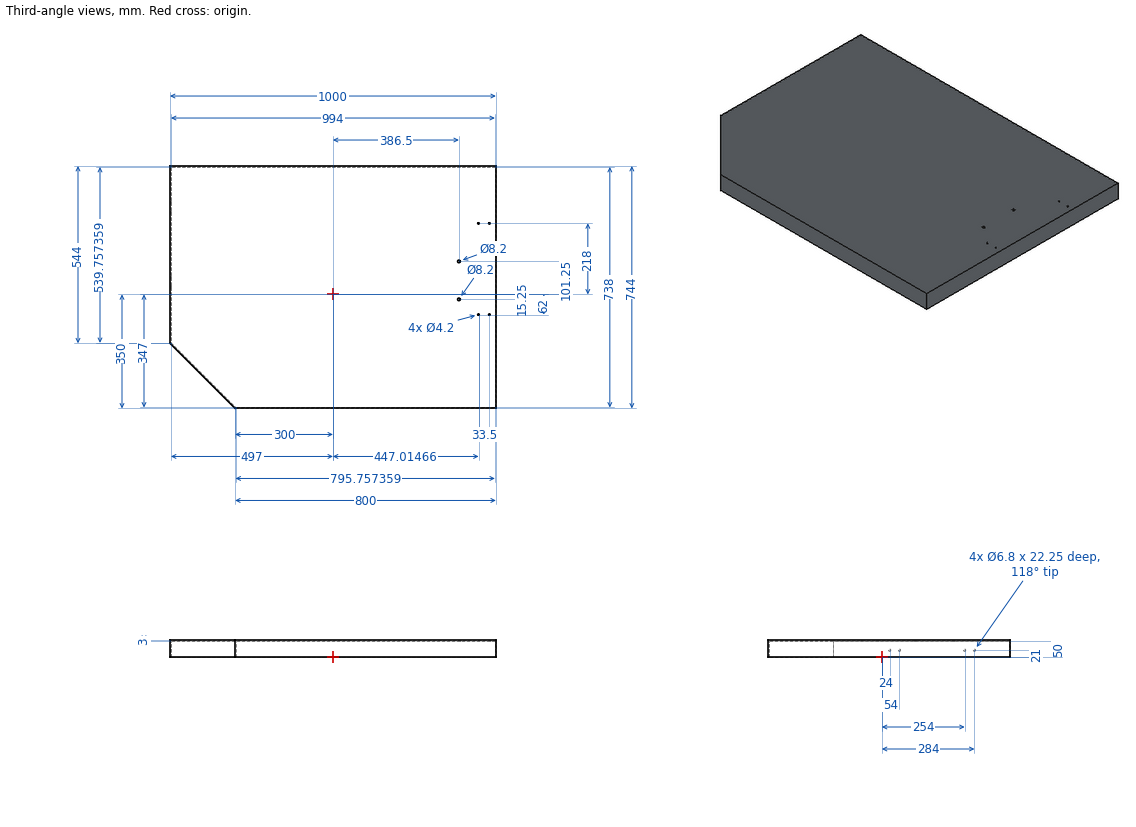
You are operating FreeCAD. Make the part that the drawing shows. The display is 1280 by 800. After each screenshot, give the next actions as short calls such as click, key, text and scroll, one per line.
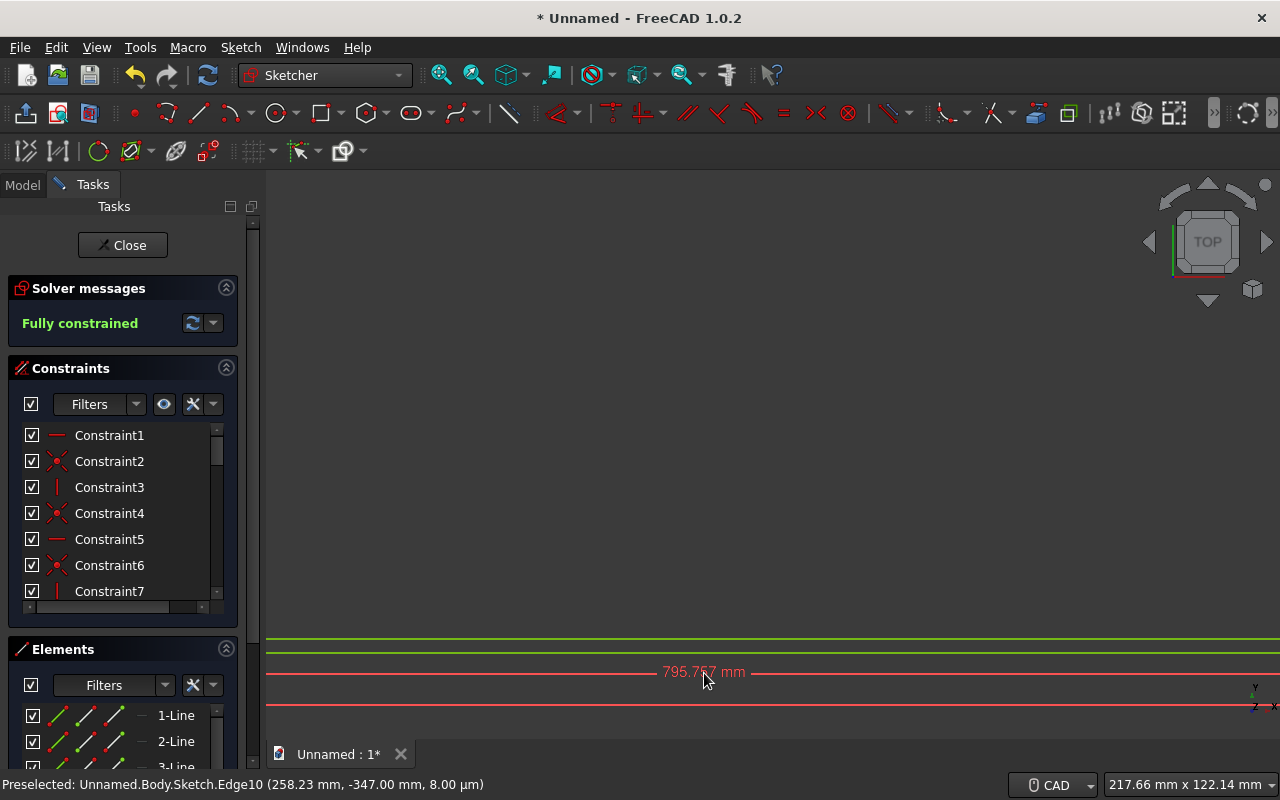
click(123, 245)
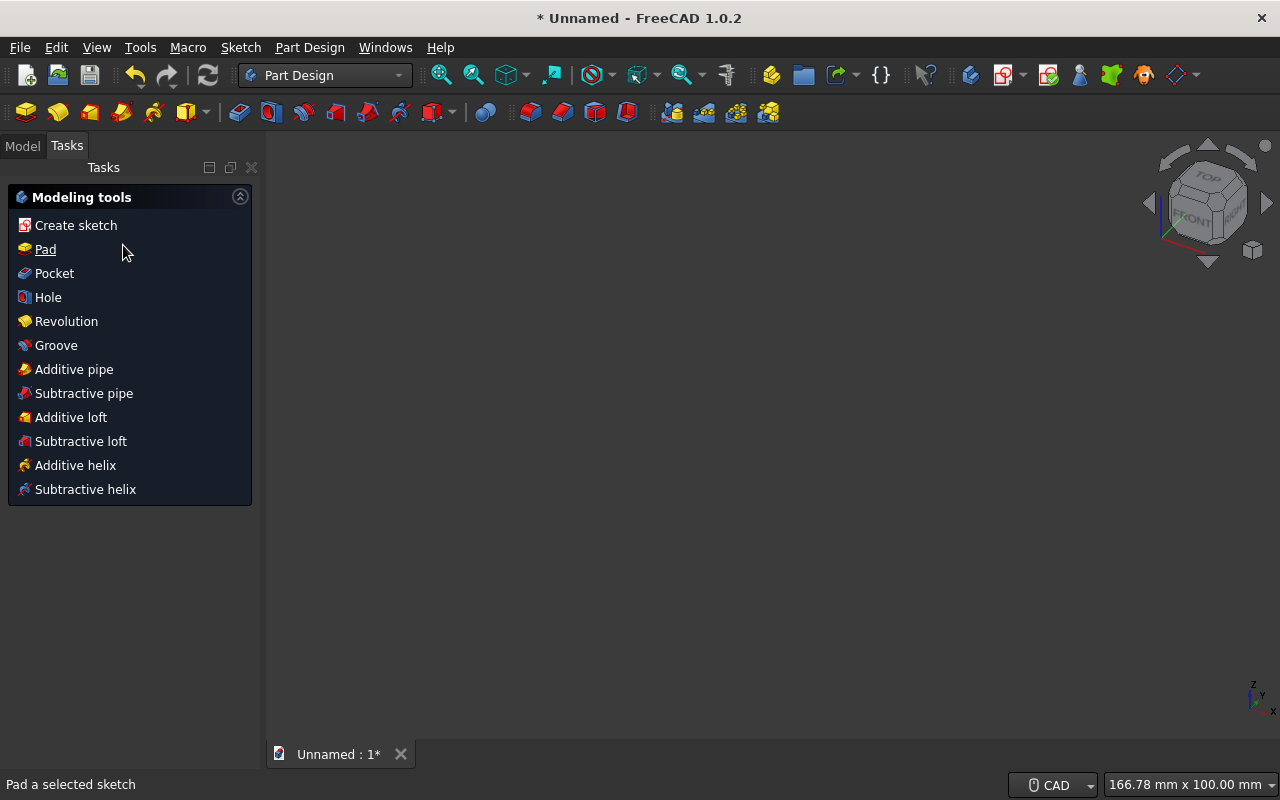
click(26, 112)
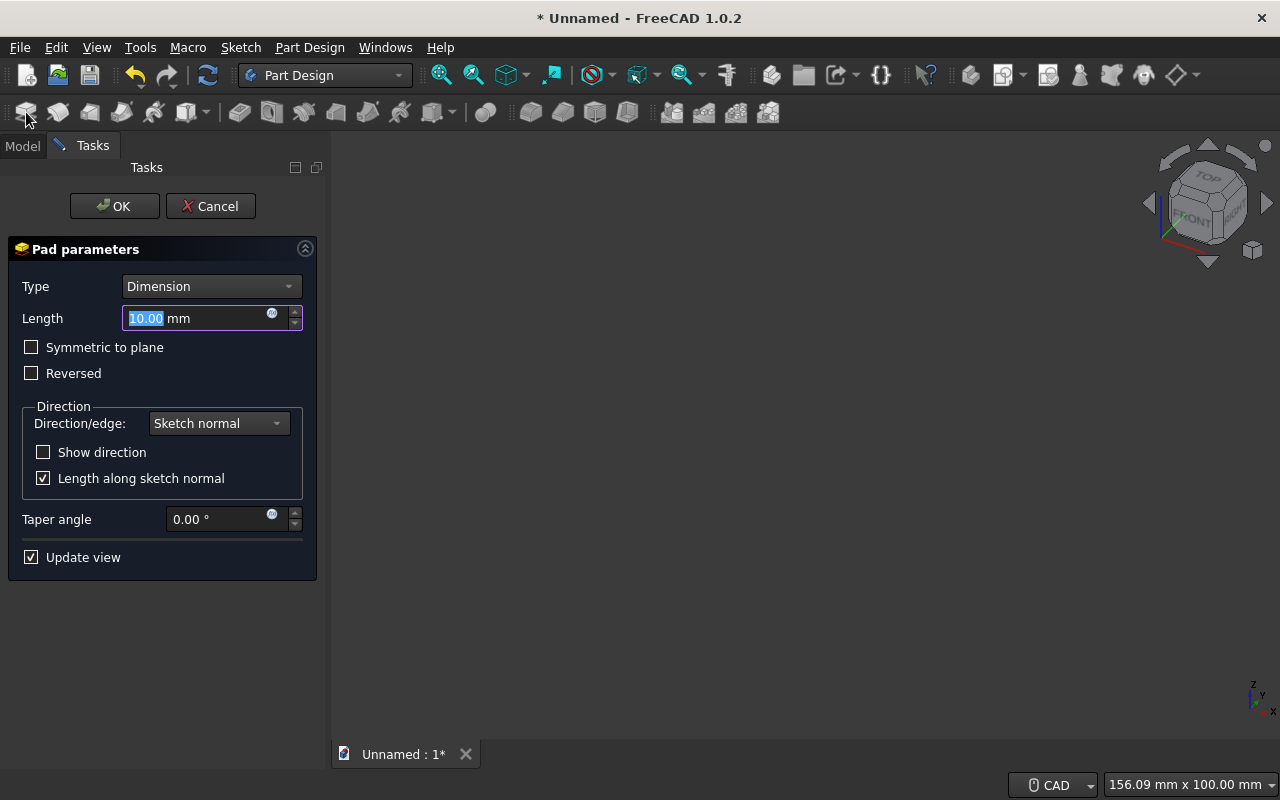
text(50)
key(Tab)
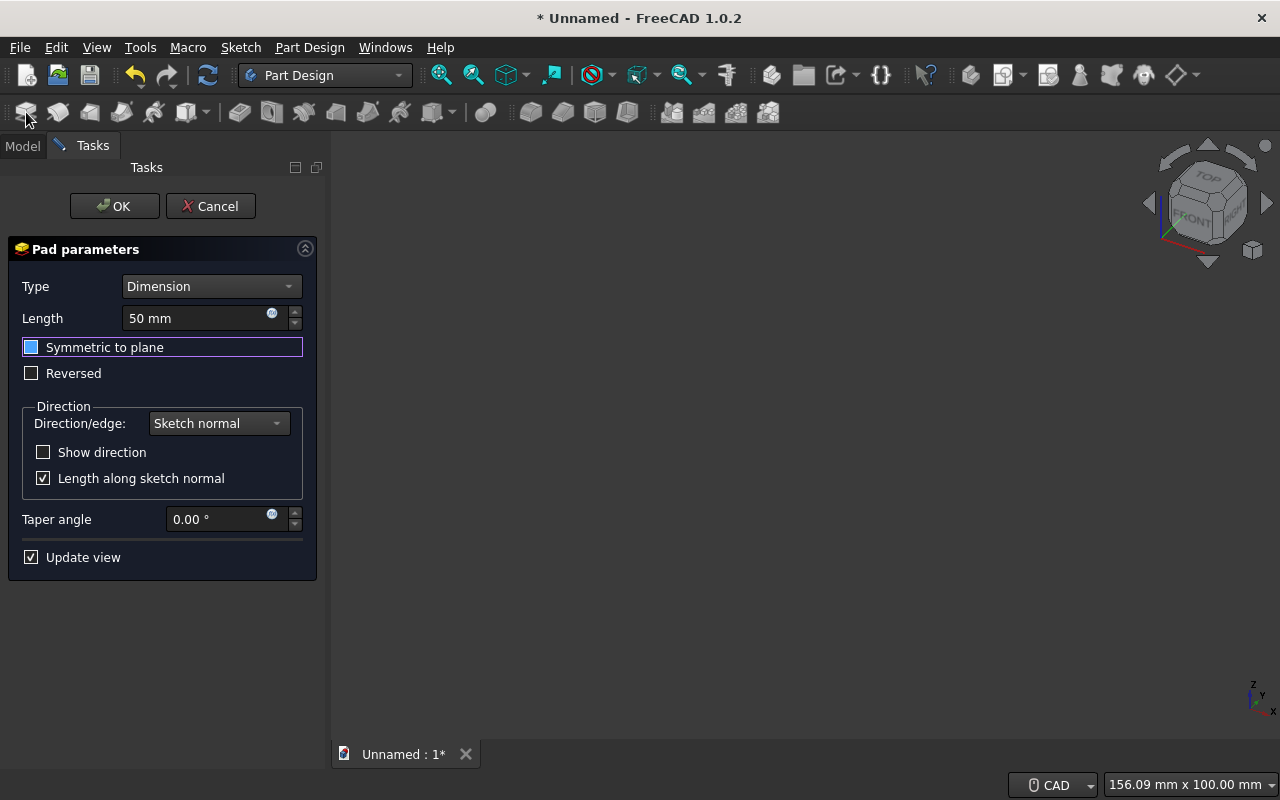
click(115, 206)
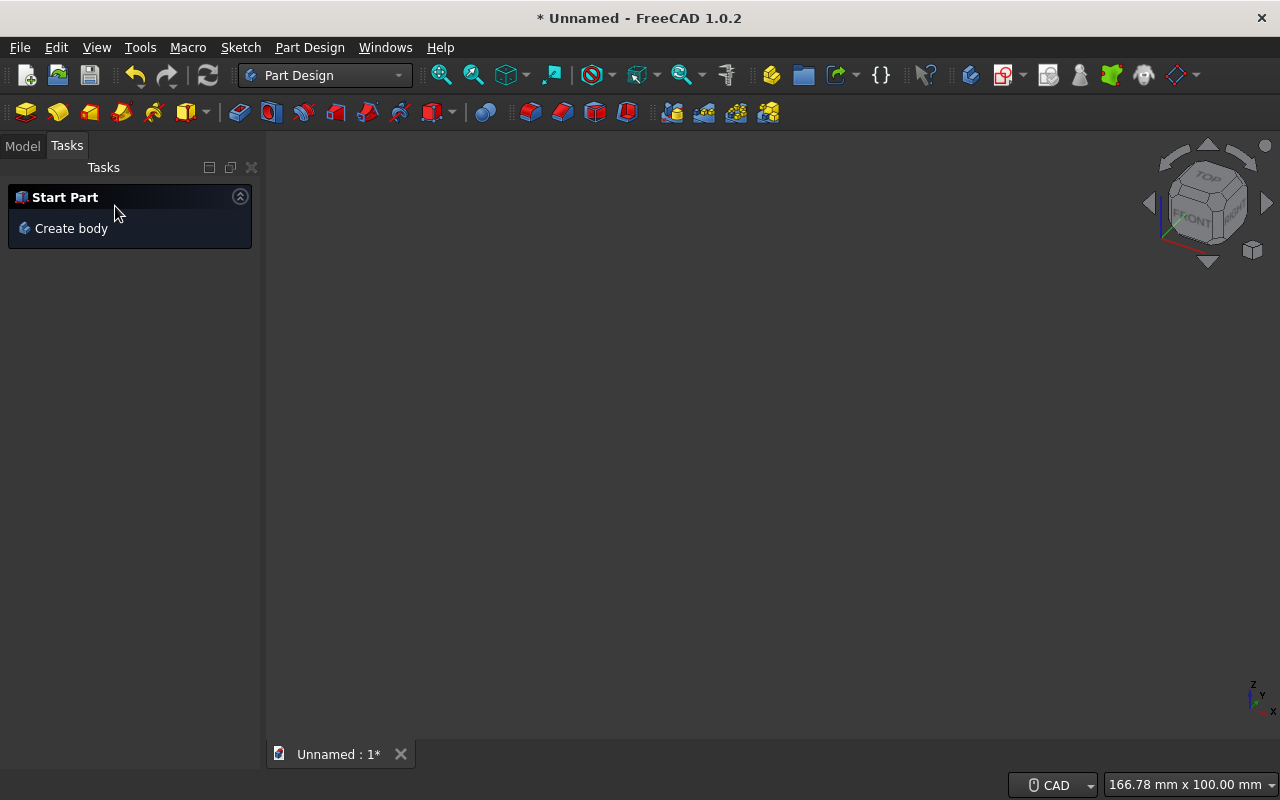
click(442, 76)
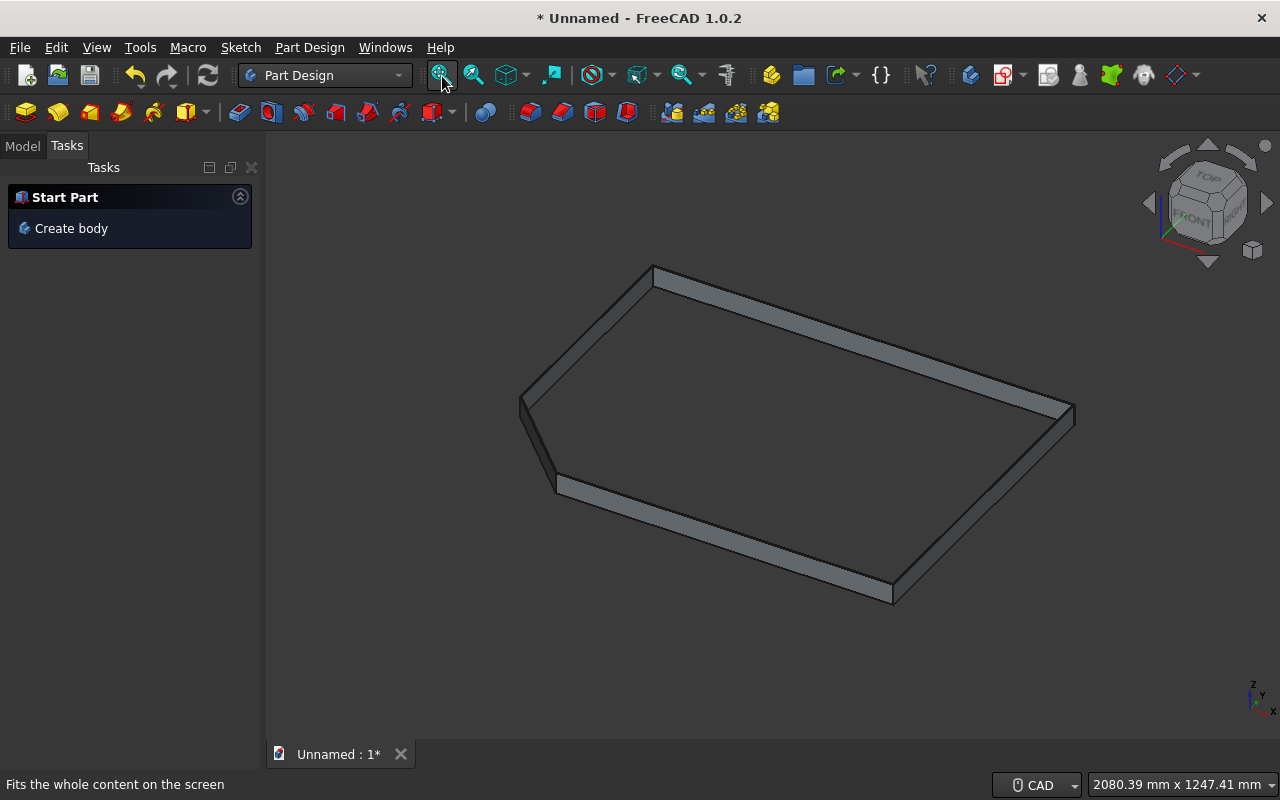
scroll(544, 447, up, 15)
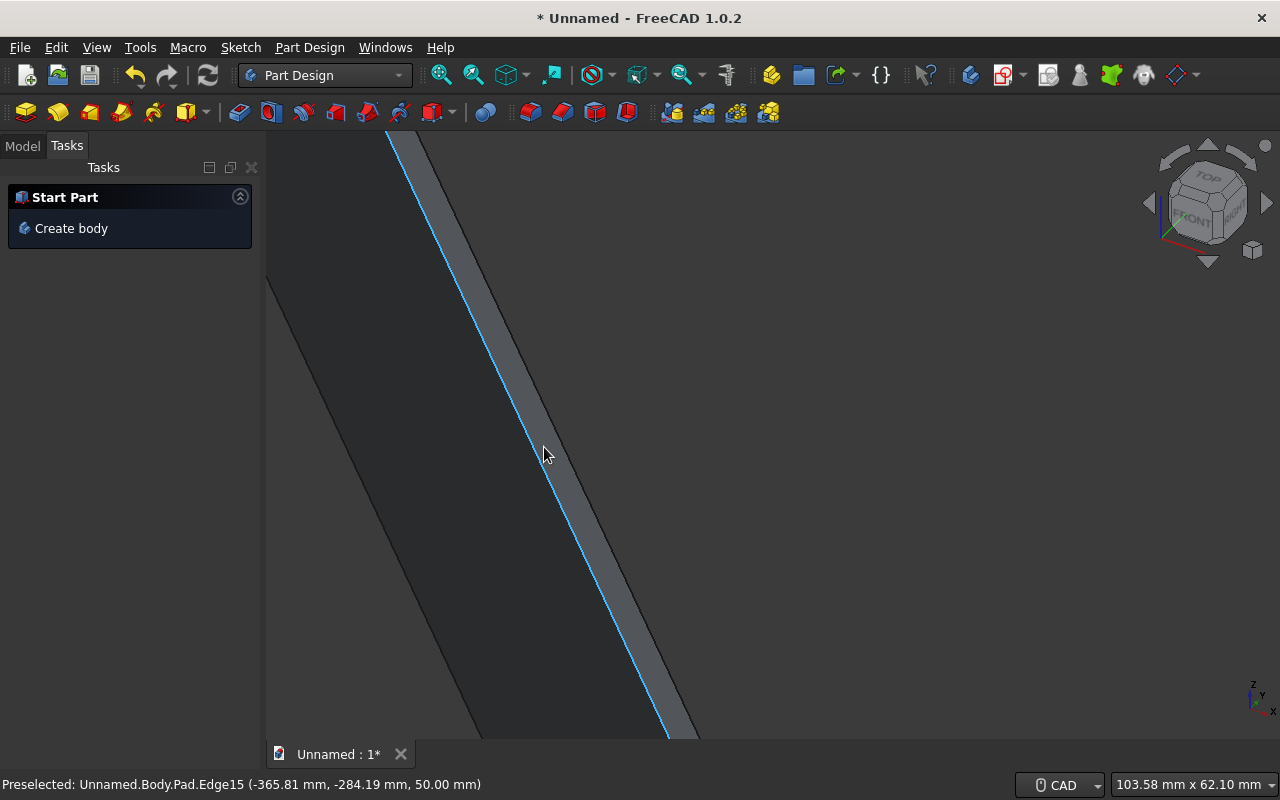
click(442, 76)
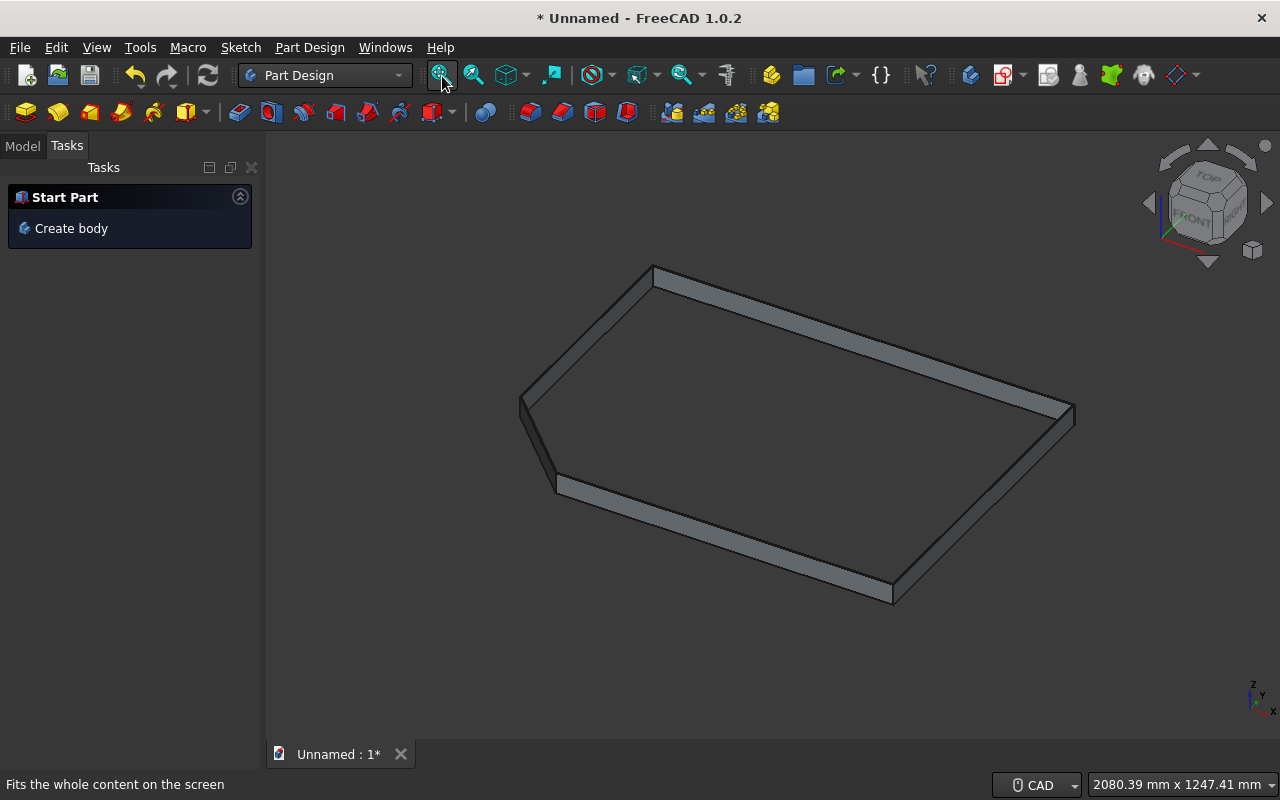
key(0)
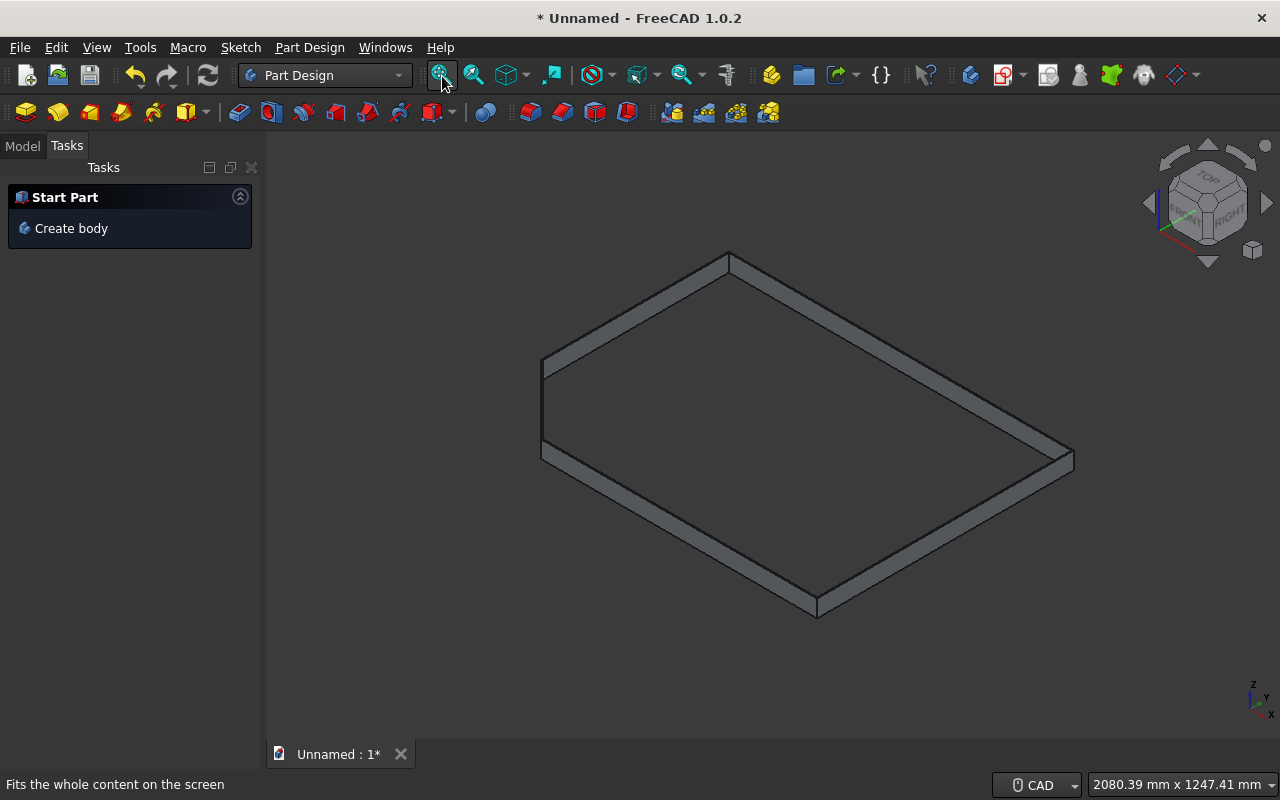
scroll(542, 412, up, 15)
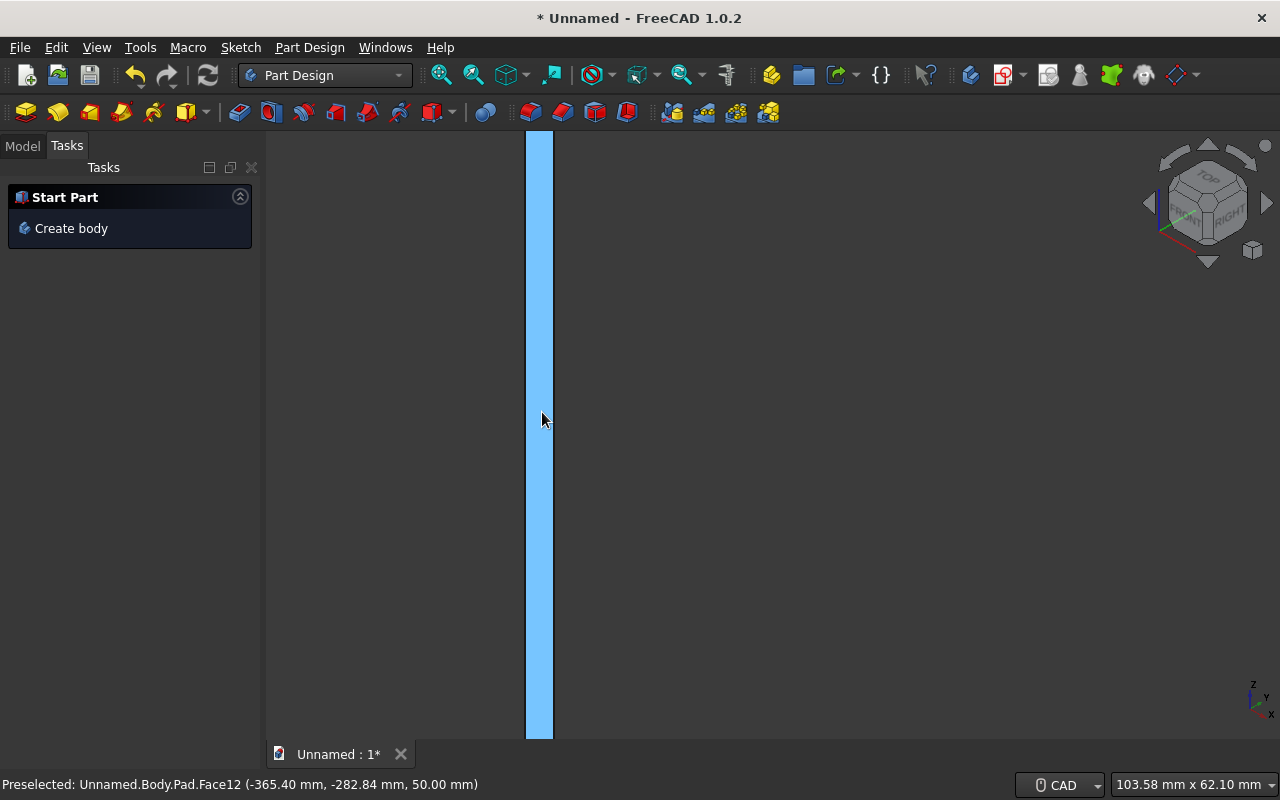
click(534, 417)